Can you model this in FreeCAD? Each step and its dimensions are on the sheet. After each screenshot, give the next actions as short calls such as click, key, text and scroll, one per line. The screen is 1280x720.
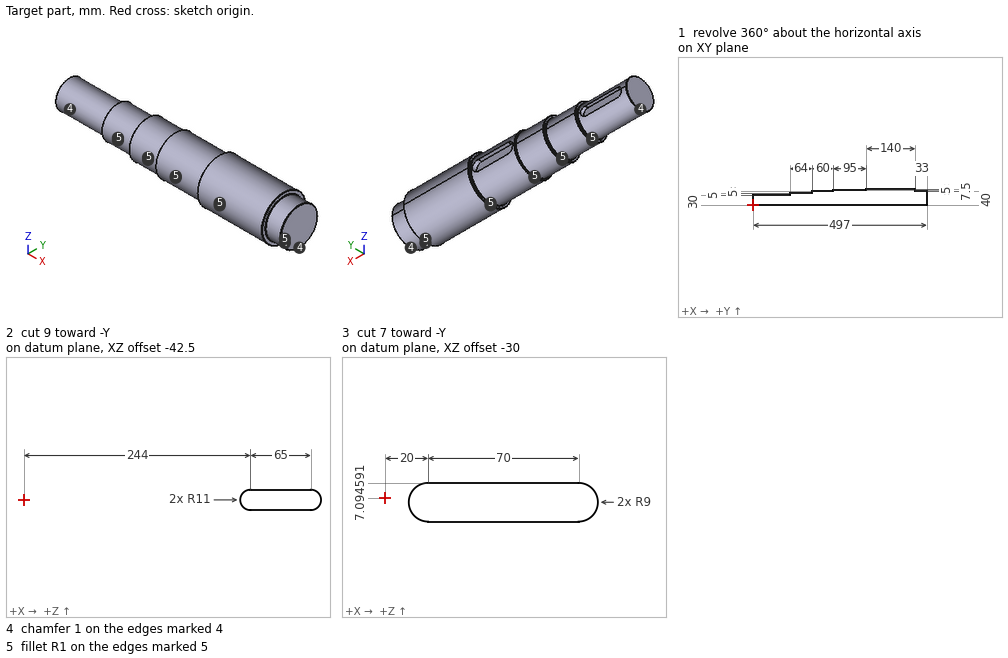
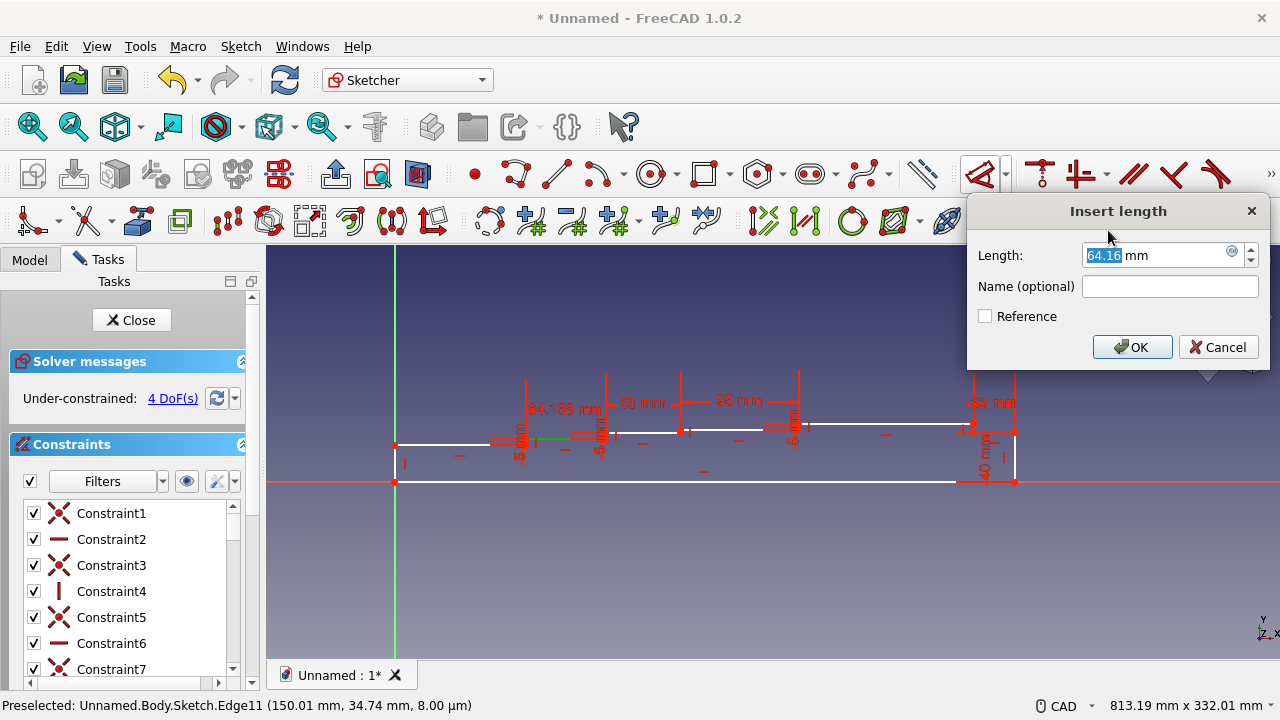
text(64)
key(Return)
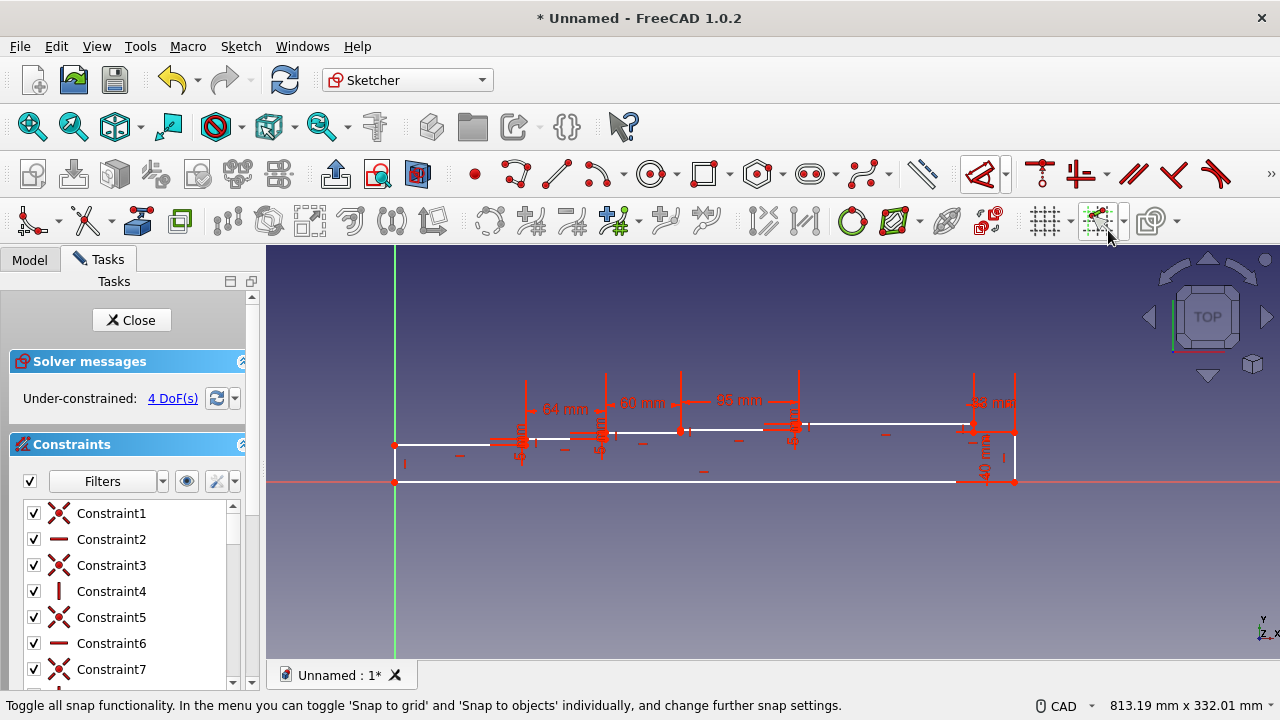
scroll(395, 456, up, 2)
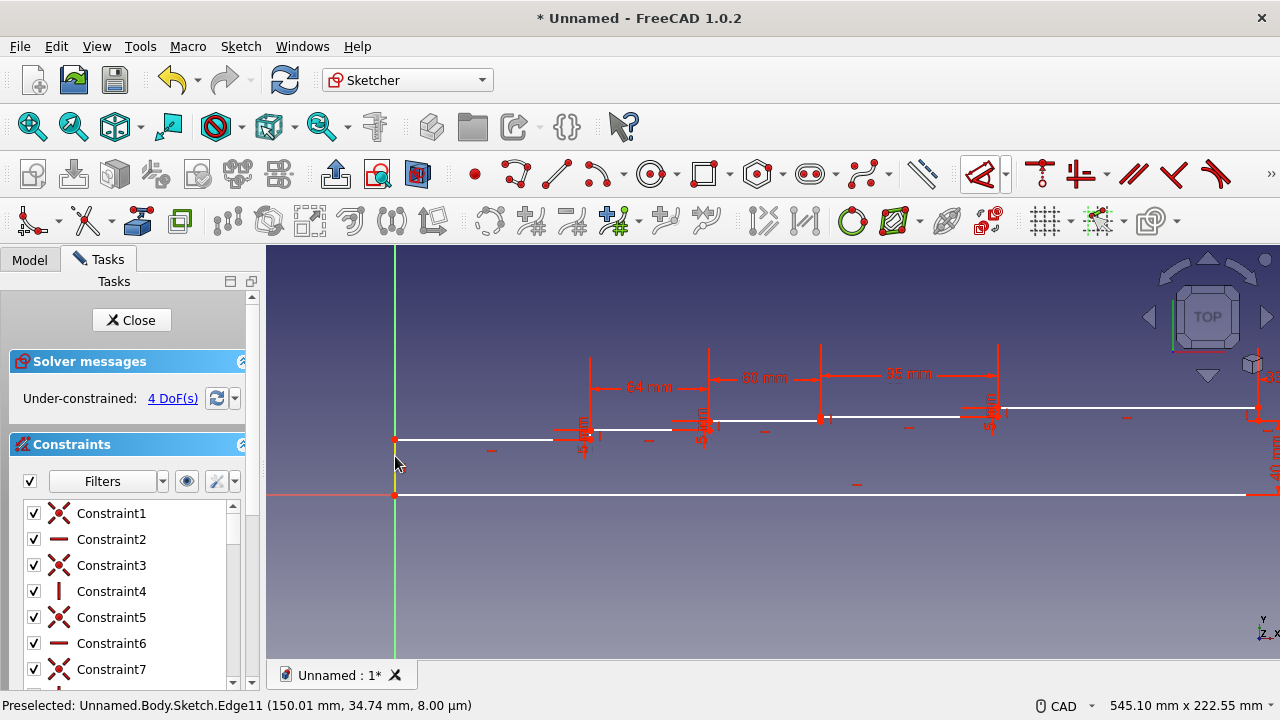
click(395, 456)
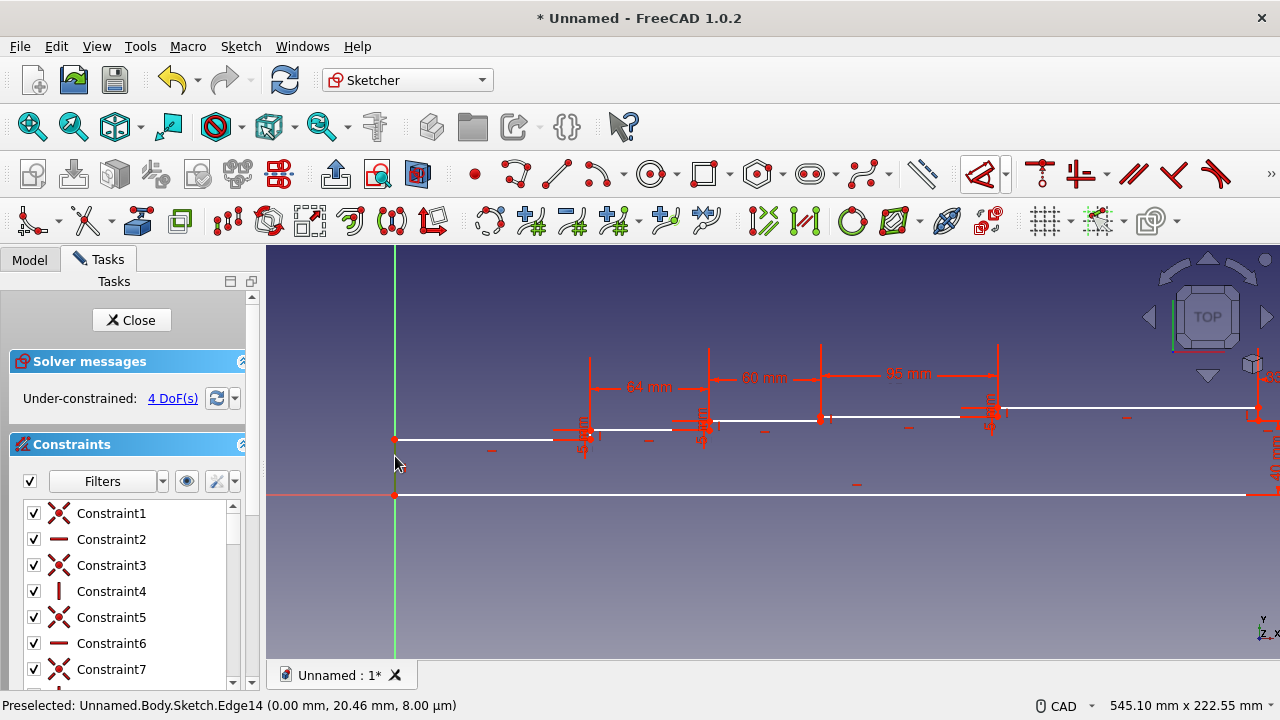
click(1006, 174)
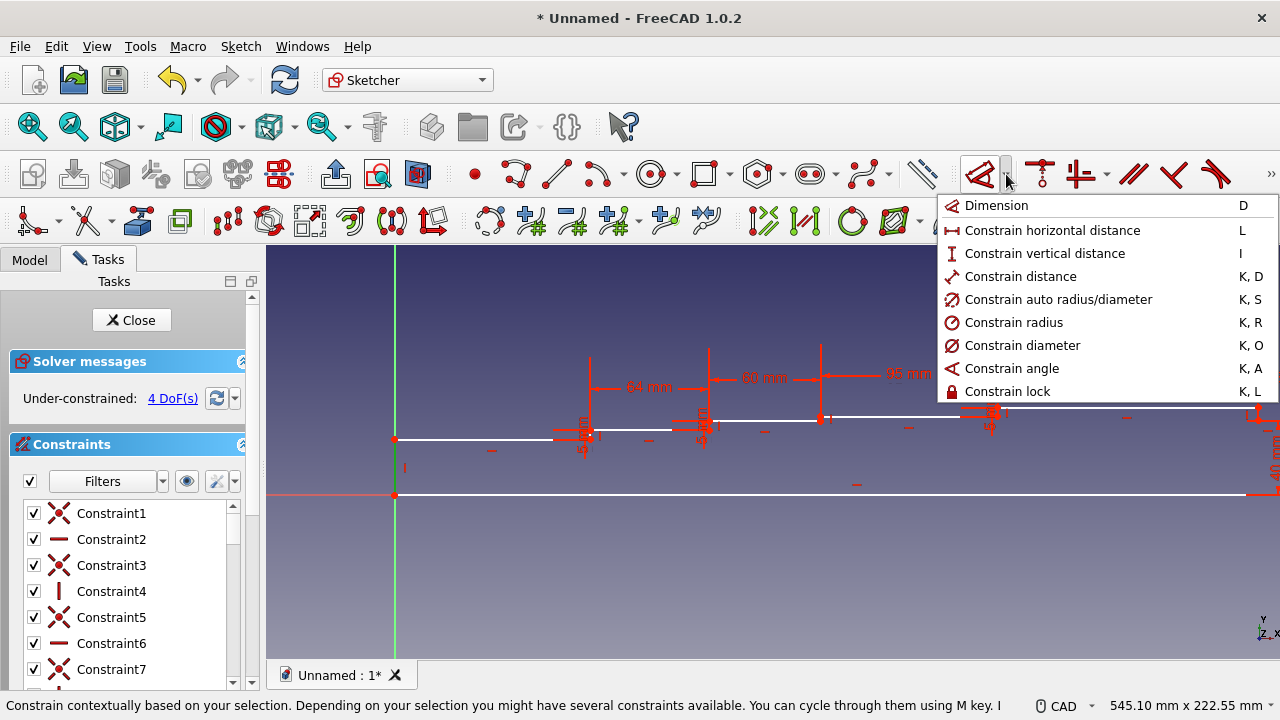
click(1108, 254)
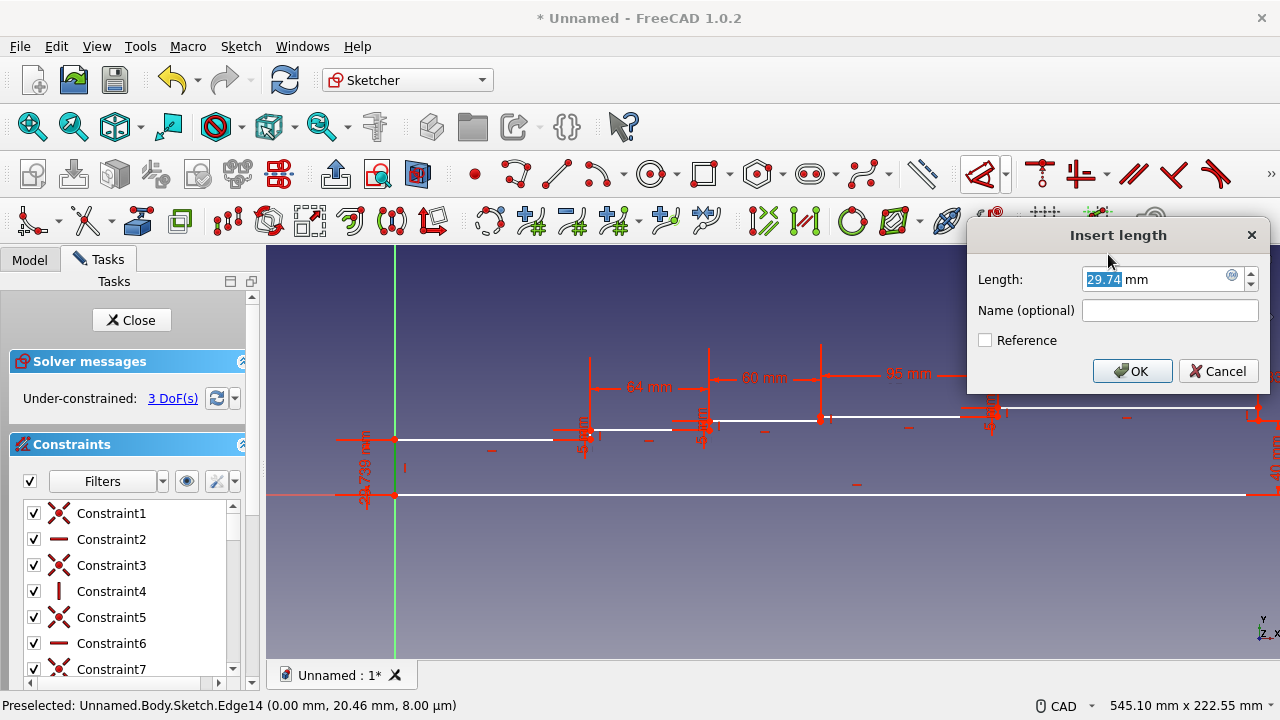
text(30)
key(Return)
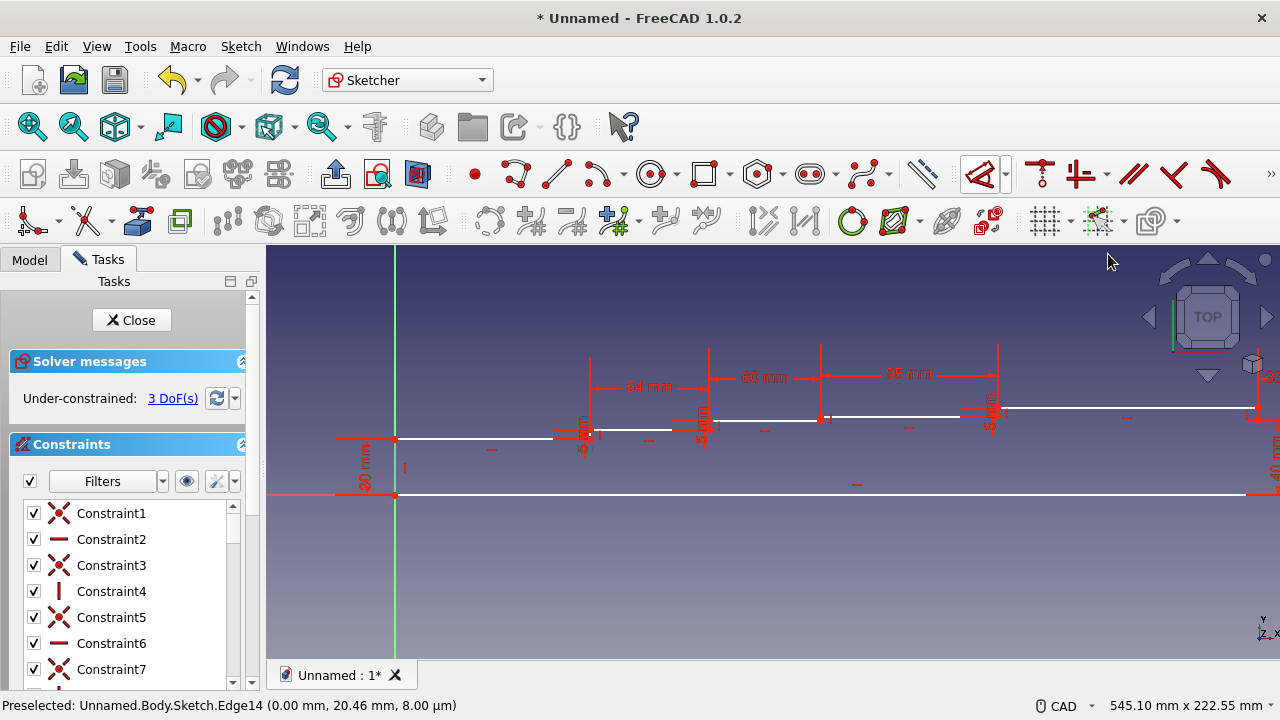
click(672, 495)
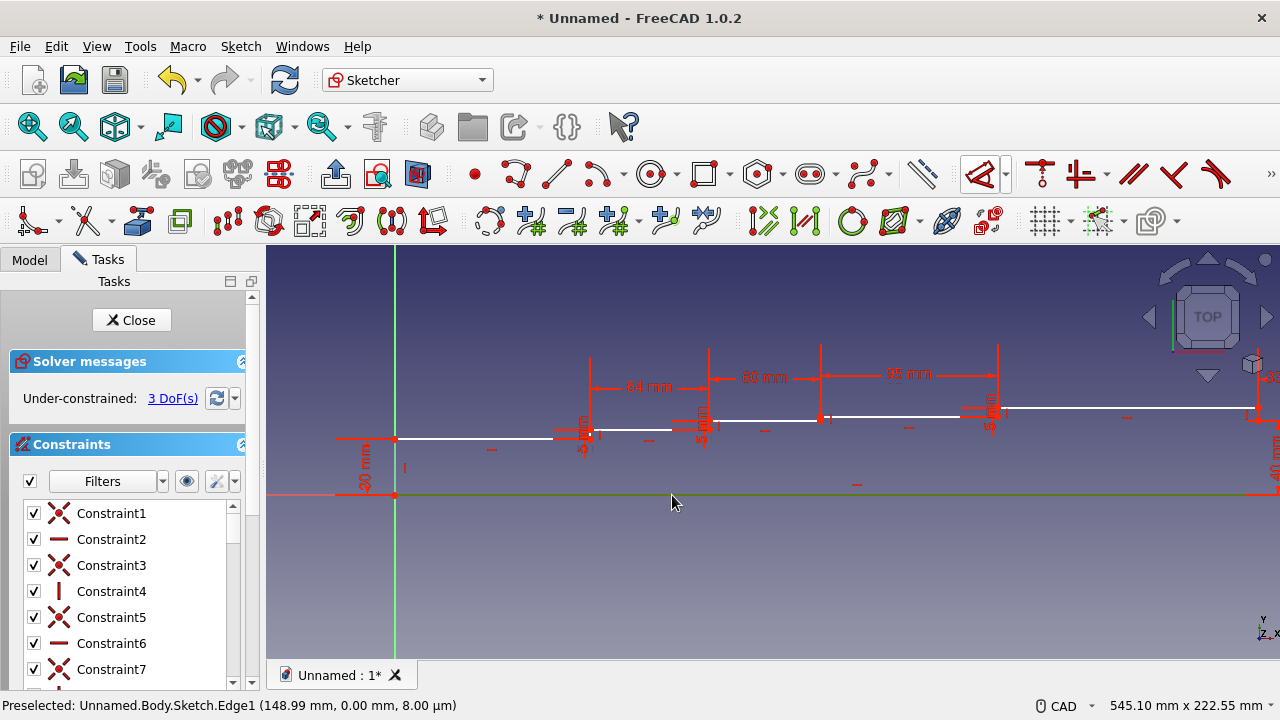
key(l)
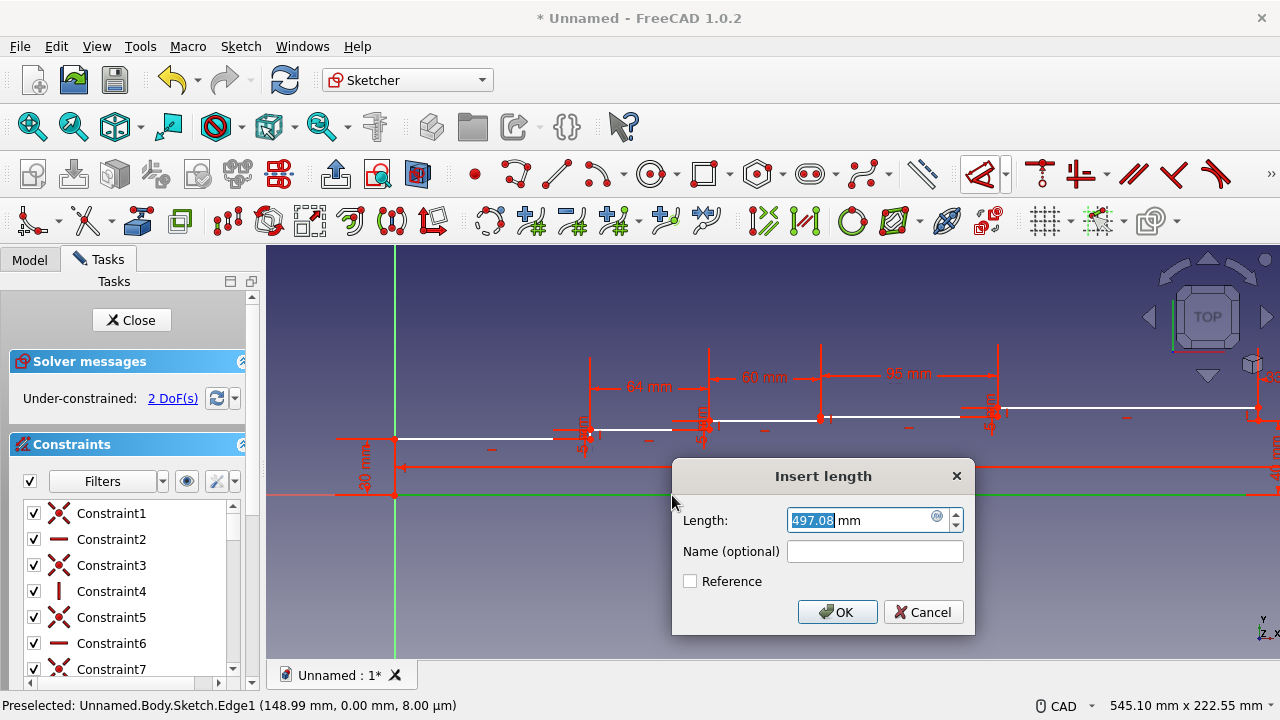
text(497)
key(Return)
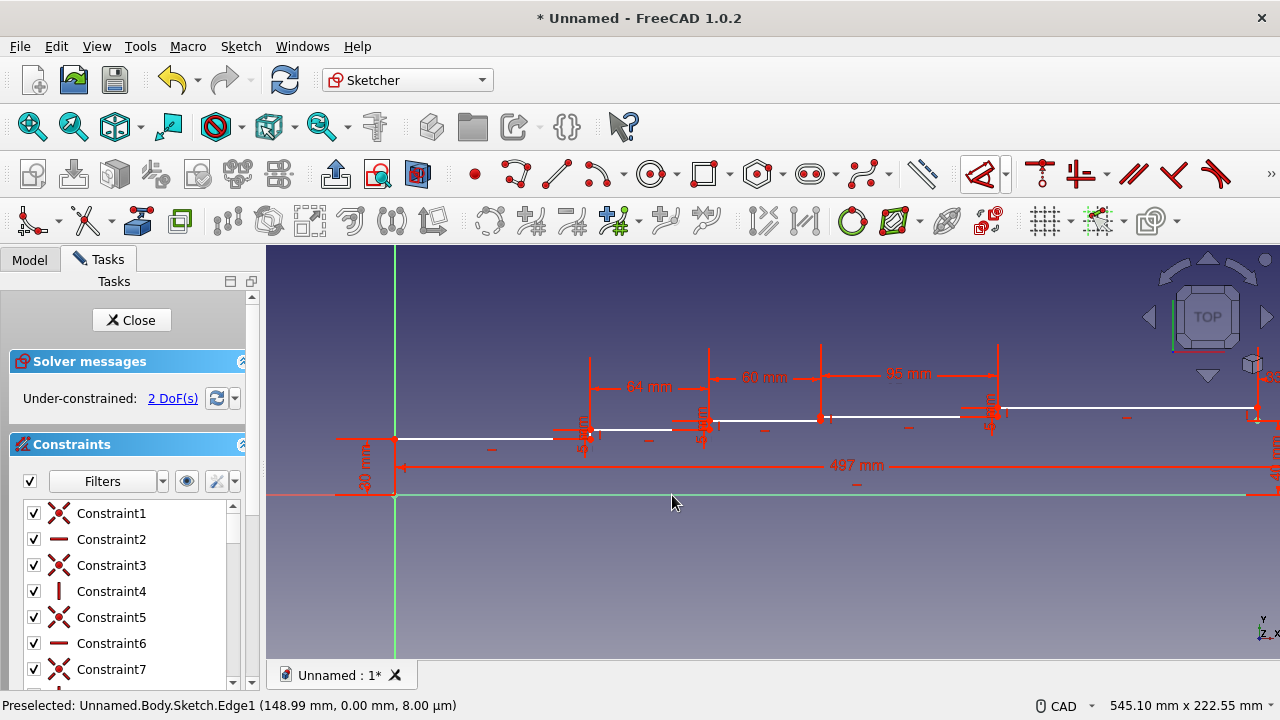
scroll(394, 454, down, 2)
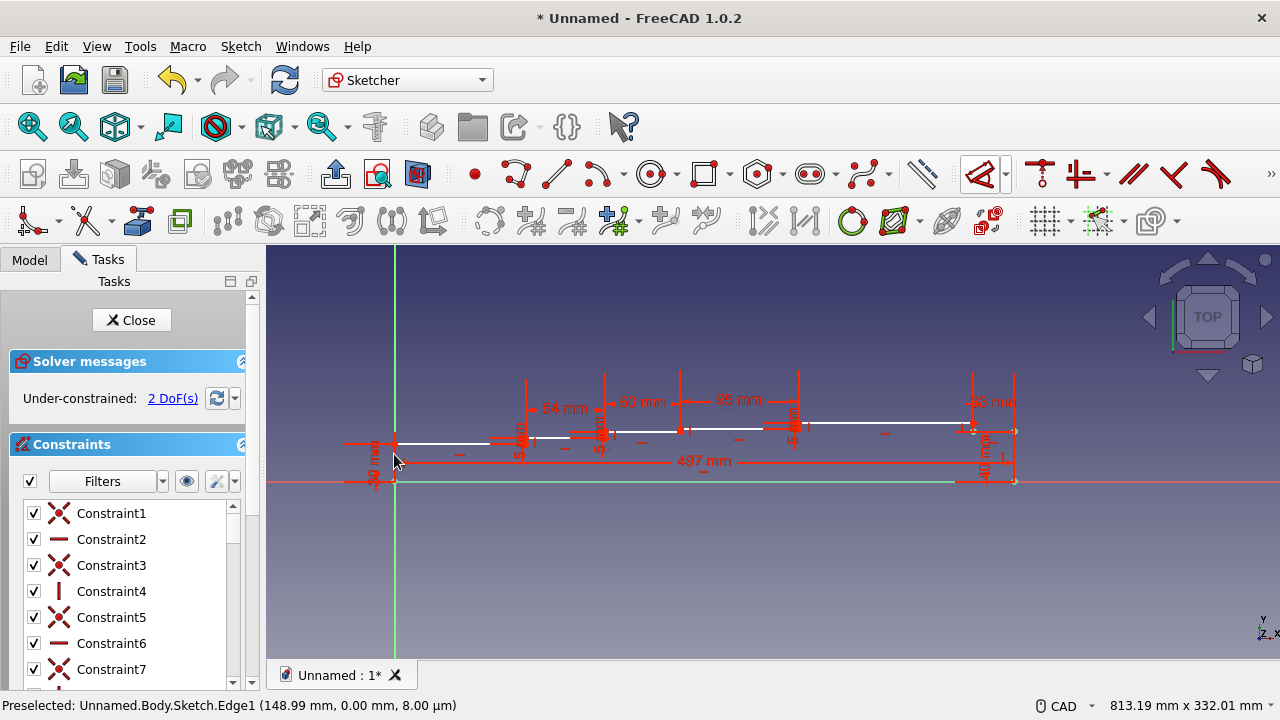
scroll(973, 427, up, 8)